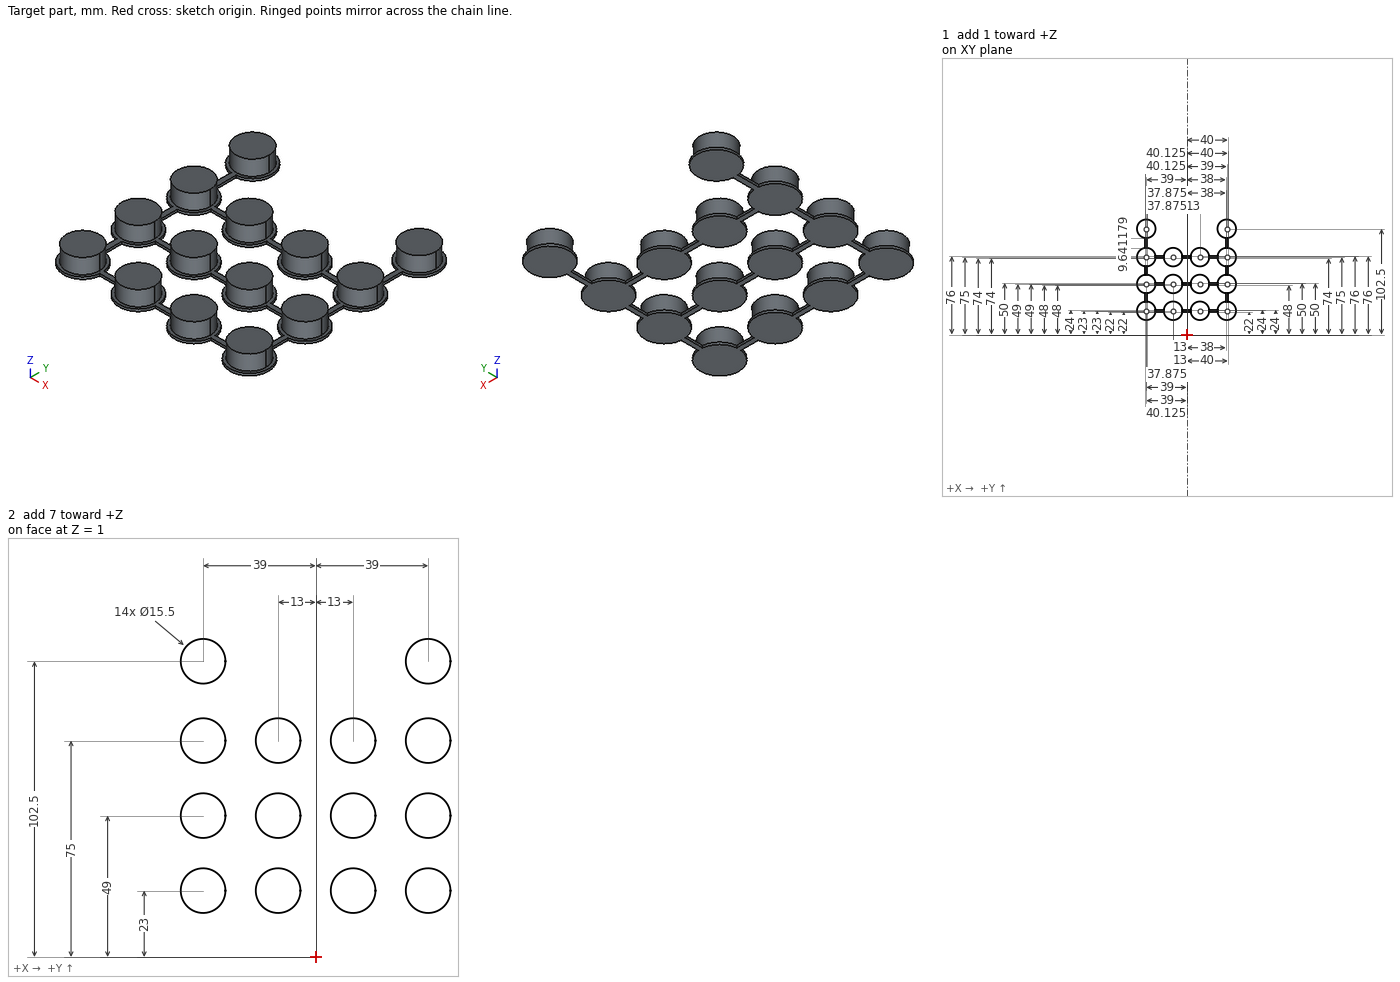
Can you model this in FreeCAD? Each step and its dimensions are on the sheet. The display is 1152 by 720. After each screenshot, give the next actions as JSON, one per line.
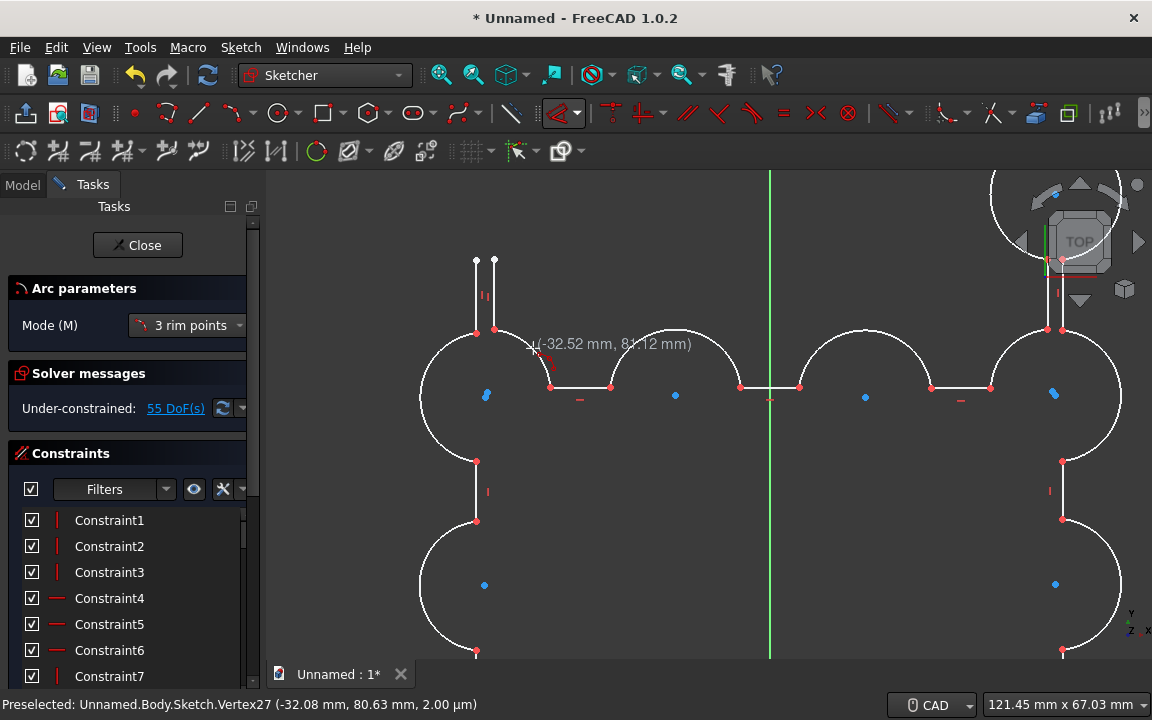
{"action": "left_click", "coordinate": [494, 259]}
{"action": "left_click", "coordinate": [476, 260]}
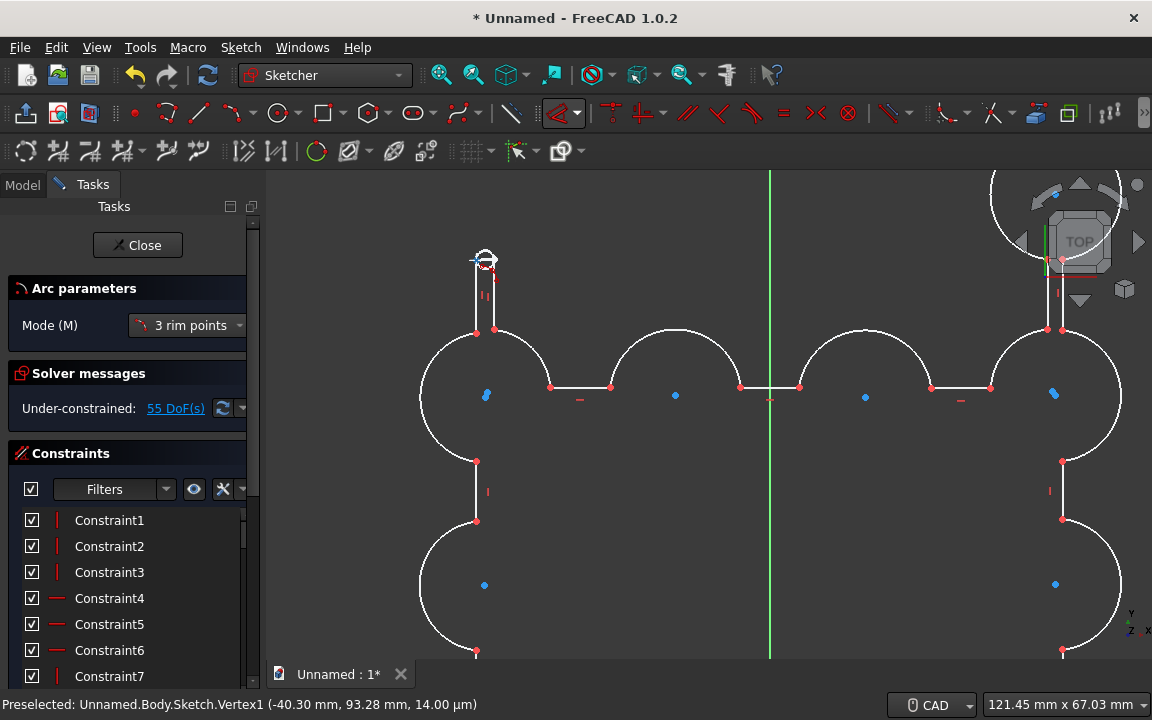
{"action": "scroll", "coordinate": [565, 345], "scroll_direction": "down", "scroll_amount": 5}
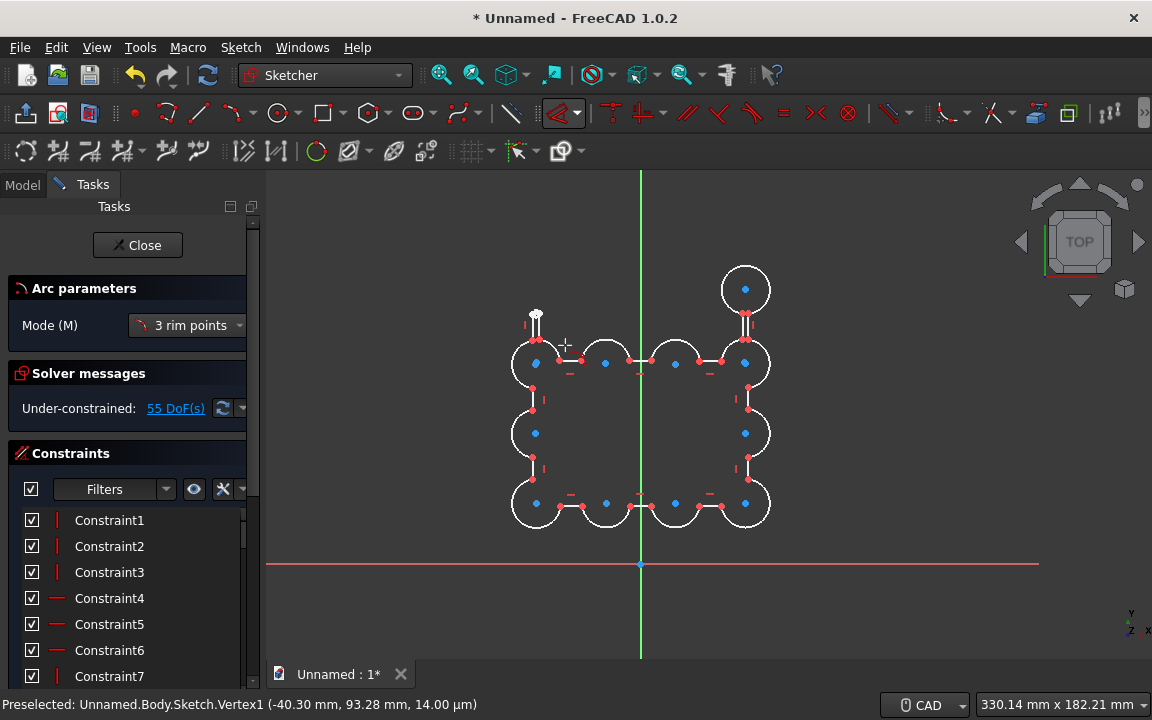
{"action": "left_click", "coordinate": [536, 265]}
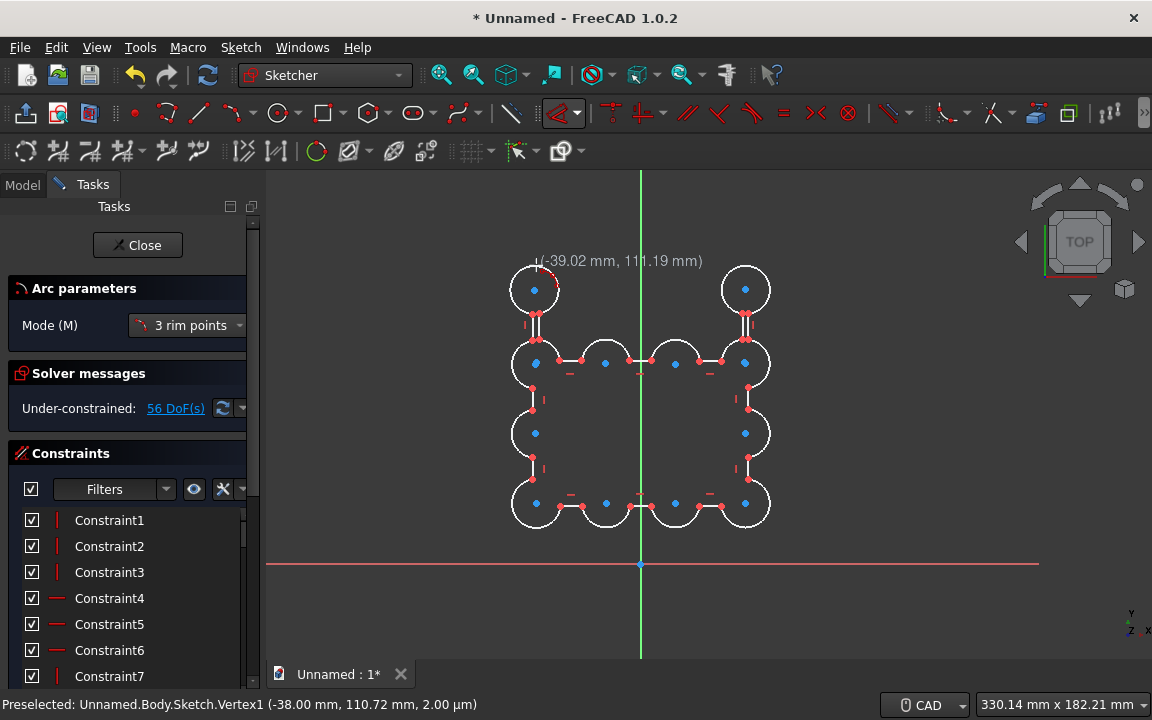
{"action": "left_click", "coordinate": [200, 114]}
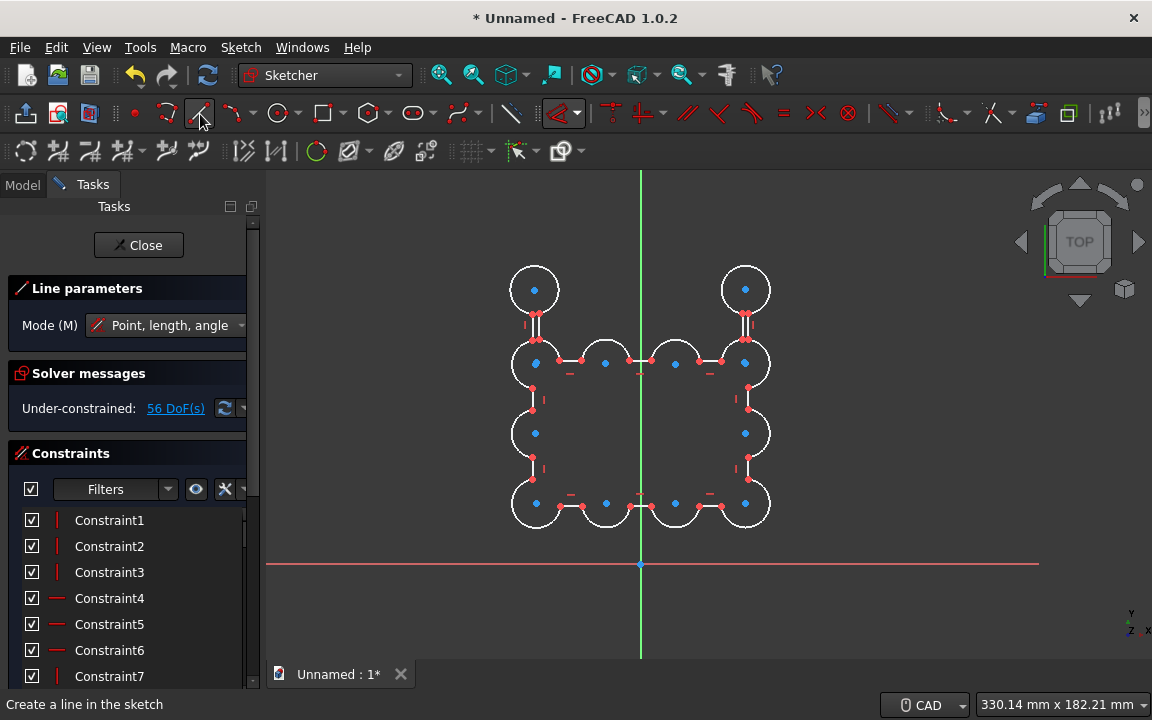
{"action": "left_click", "coordinate": [560, 436]}
{"action": "left_click", "coordinate": [582, 436]}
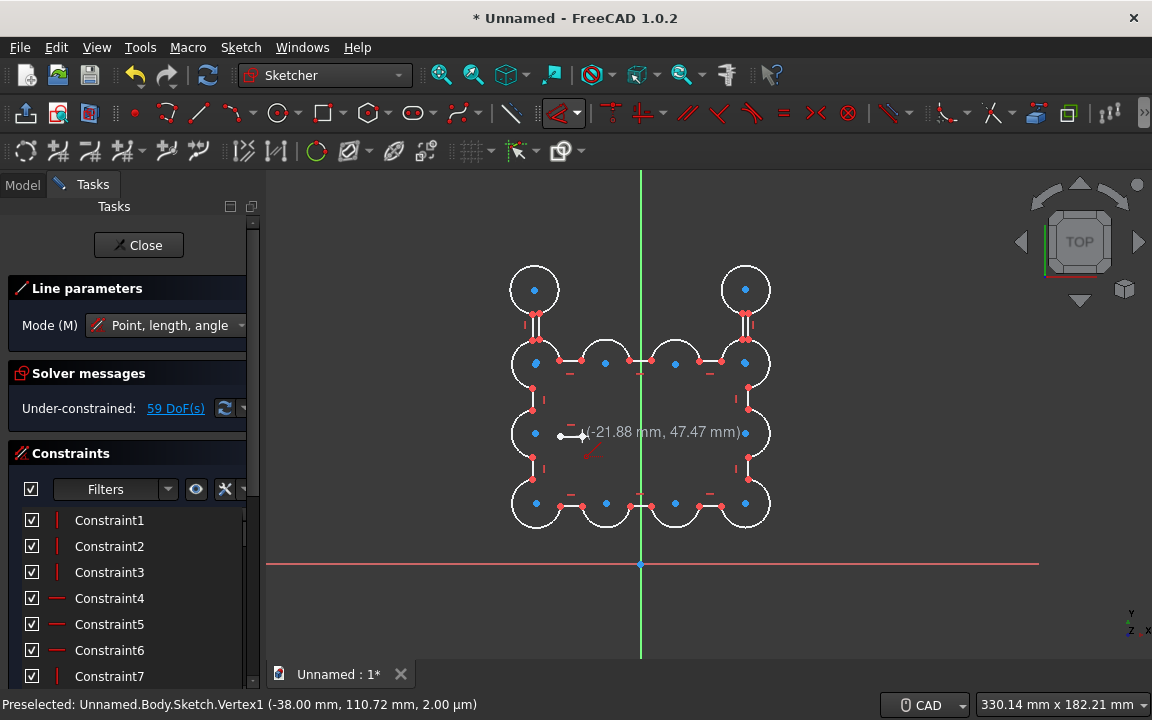
{"action": "scroll", "coordinate": [630, 436], "scroll_direction": "up", "scroll_amount": 2}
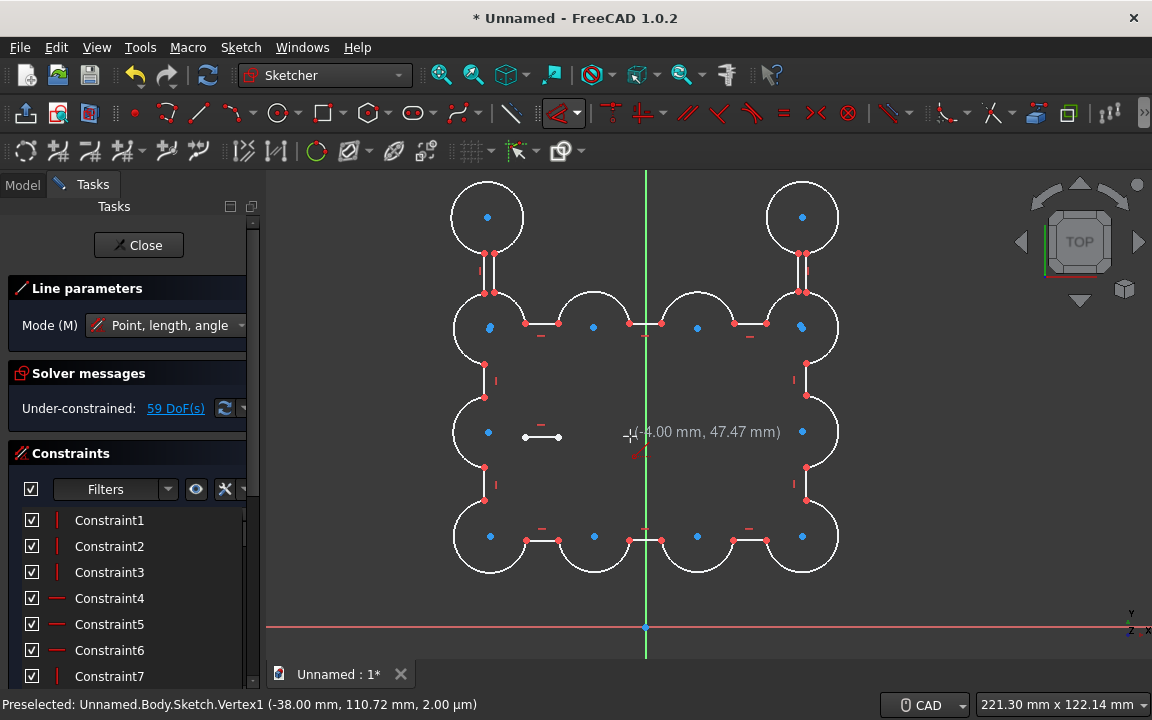
{"action": "left_click", "coordinate": [630, 435]}
{"action": "left_click", "coordinate": [662, 435]}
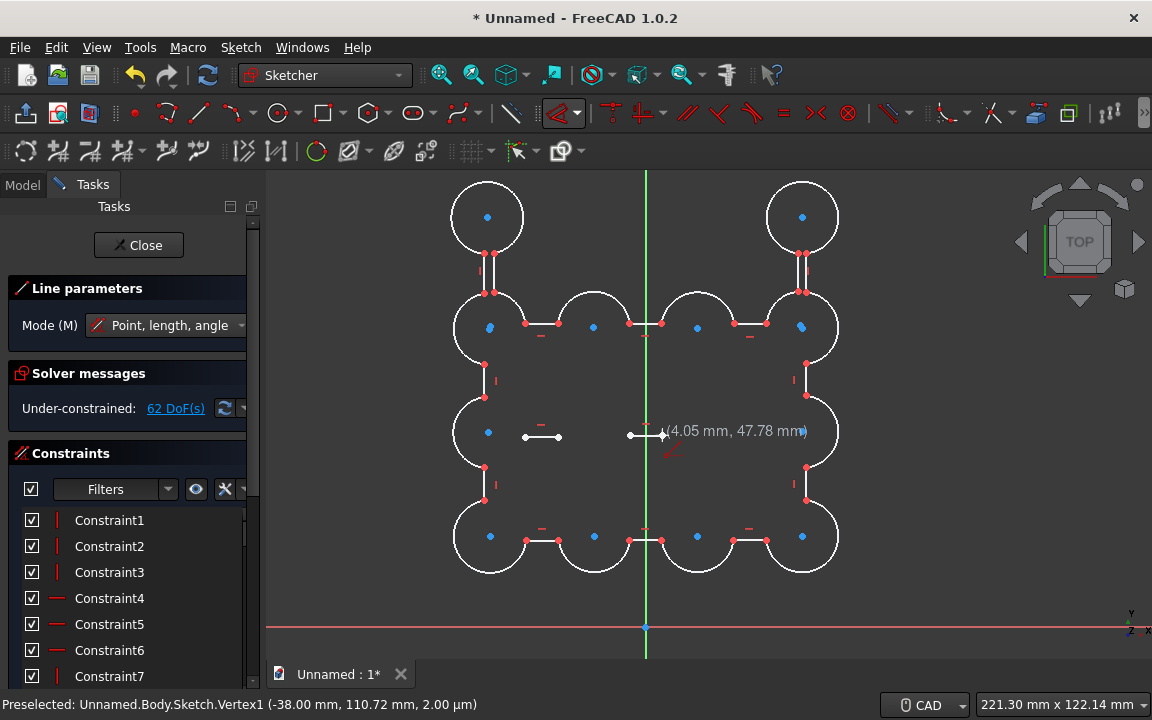
{"action": "left_click", "coordinate": [734, 435]}
{"action": "left_click", "coordinate": [766, 435]}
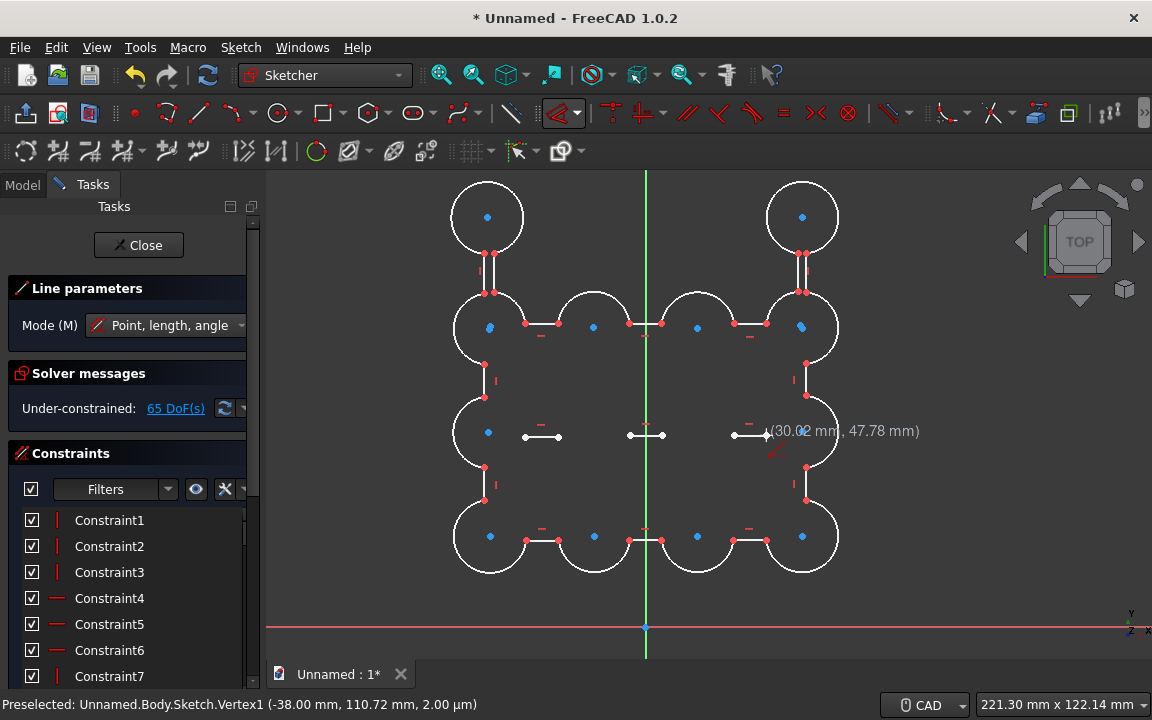
{"action": "scroll", "coordinate": [798, 467], "scroll_direction": "up", "scroll_amount": 4}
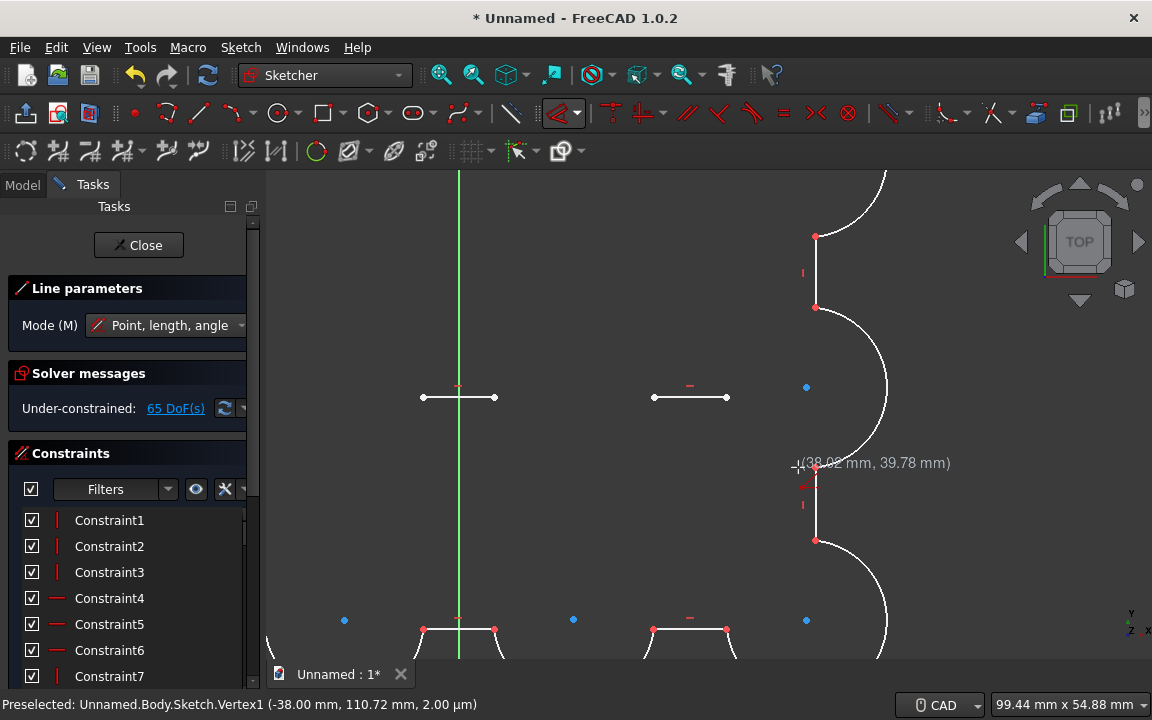
{"action": "left_click", "coordinate": [797, 466]}
{"action": "left_click", "coordinate": [797, 538]}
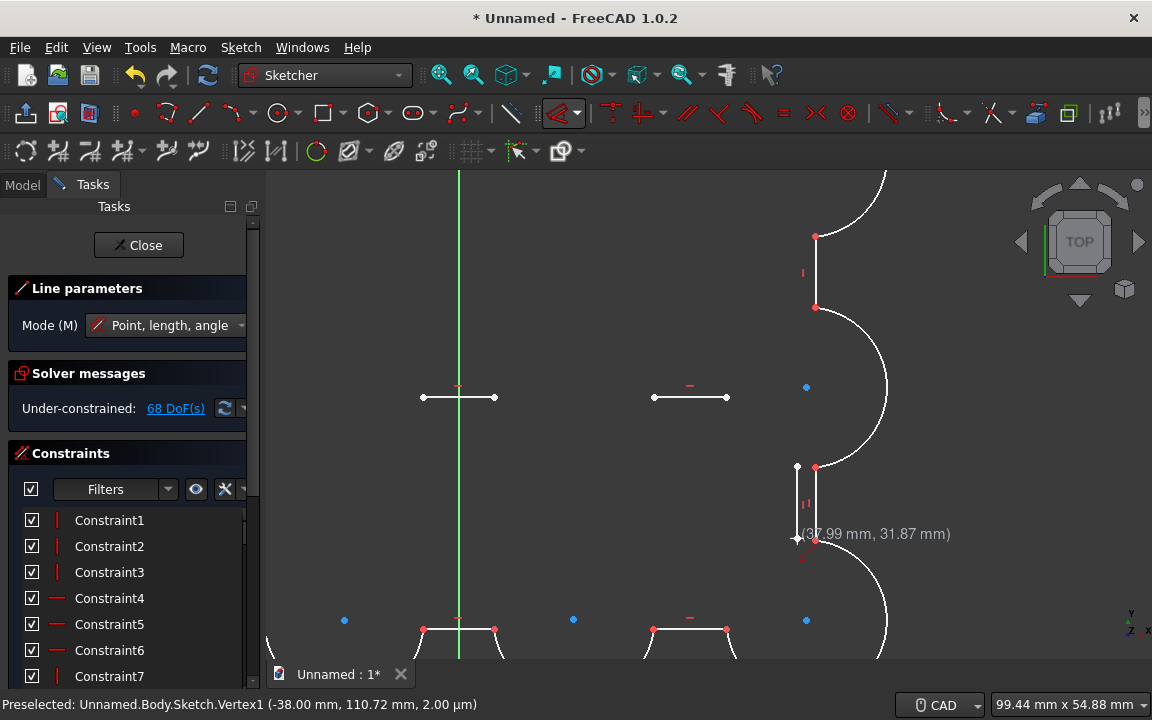
{"action": "left_click", "coordinate": [726, 609]}
{"action": "left_click", "coordinate": [654, 609]}